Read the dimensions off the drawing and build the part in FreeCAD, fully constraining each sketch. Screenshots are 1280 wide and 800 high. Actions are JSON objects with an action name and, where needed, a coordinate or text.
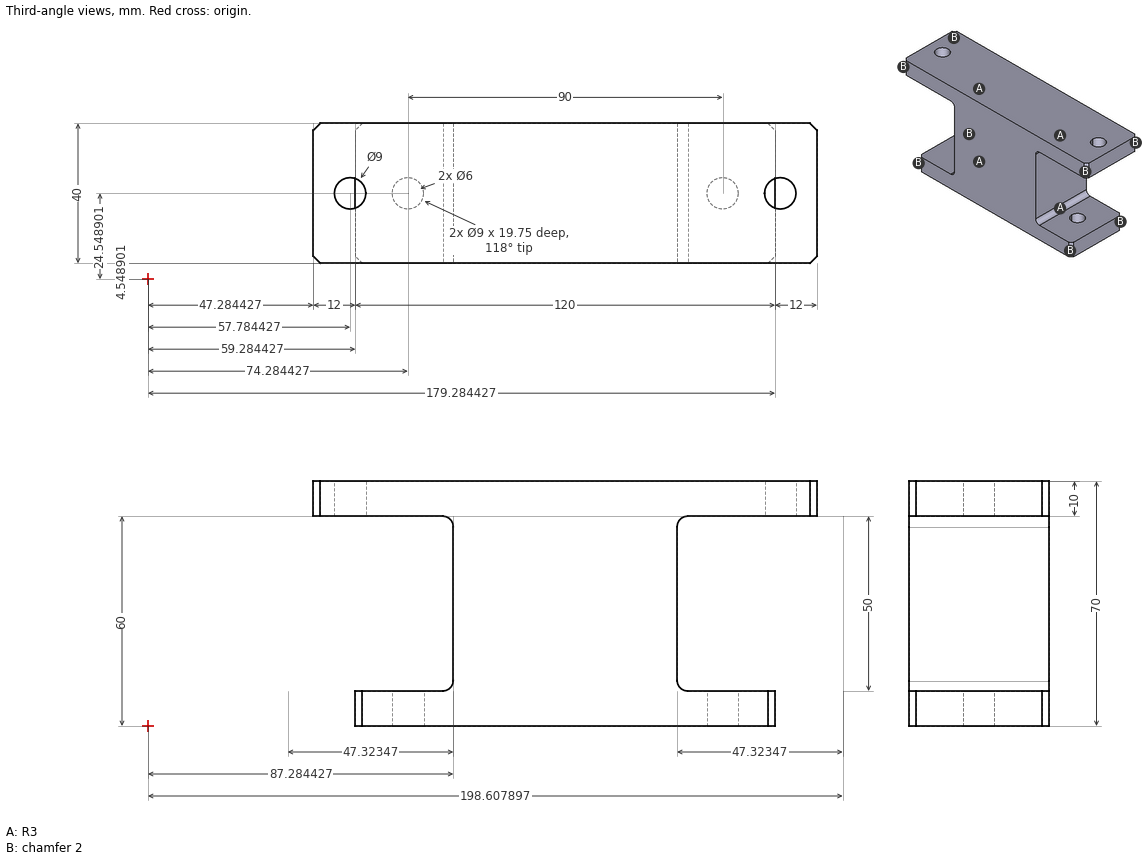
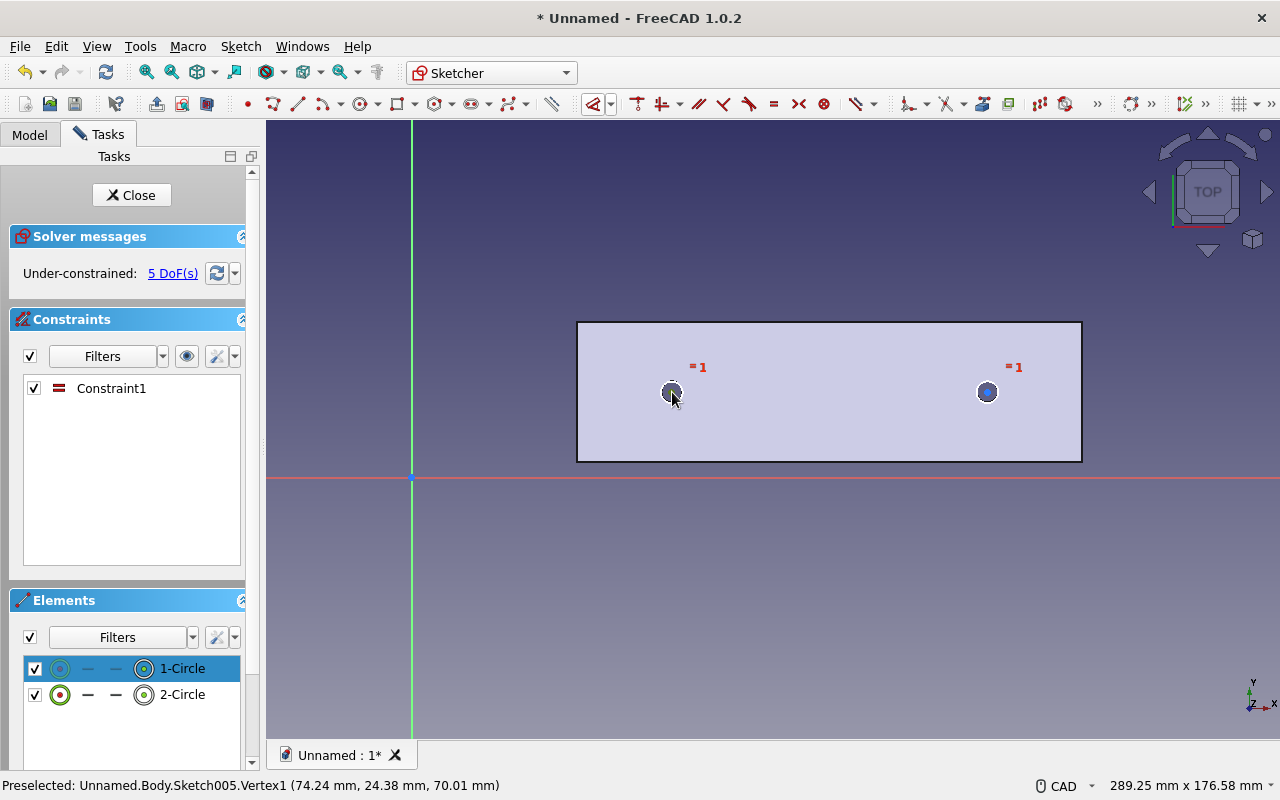
{"action": "left_click", "coordinate": [987, 392]}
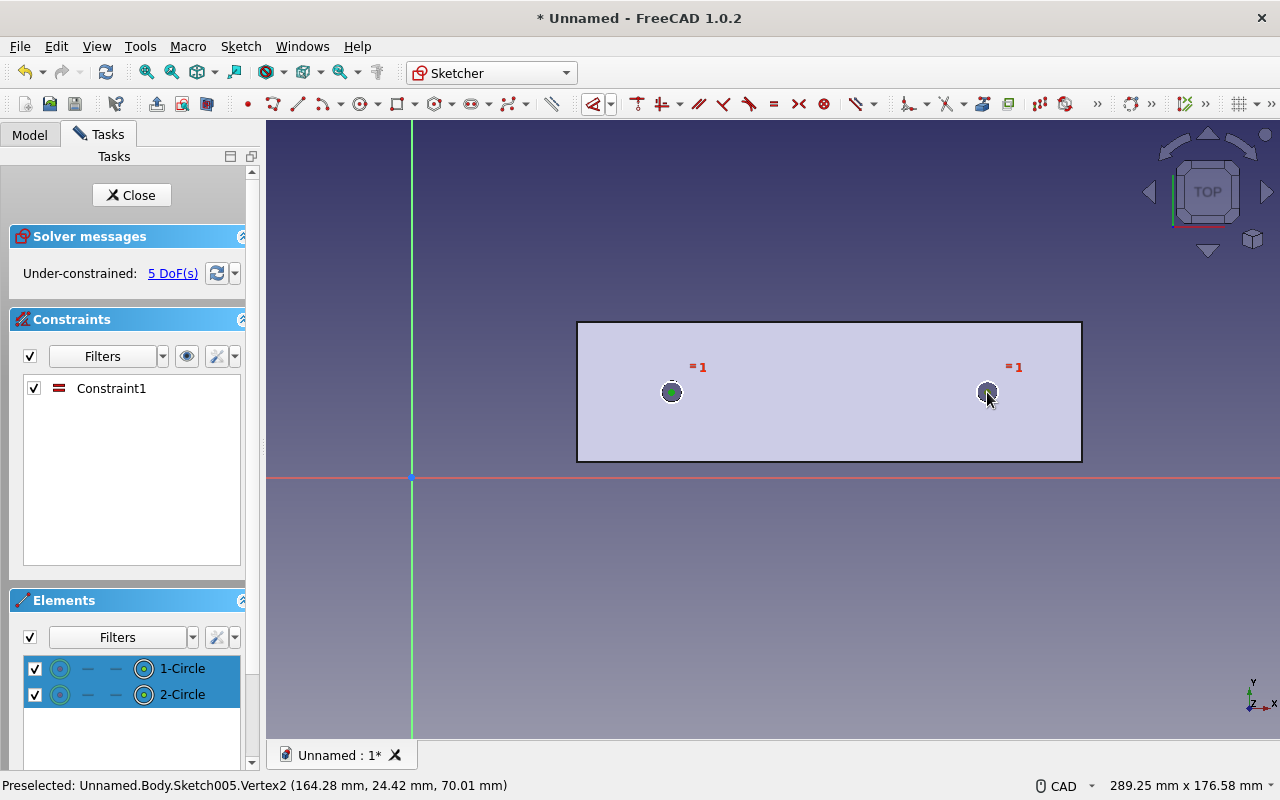
{"action": "key", "text": "h"}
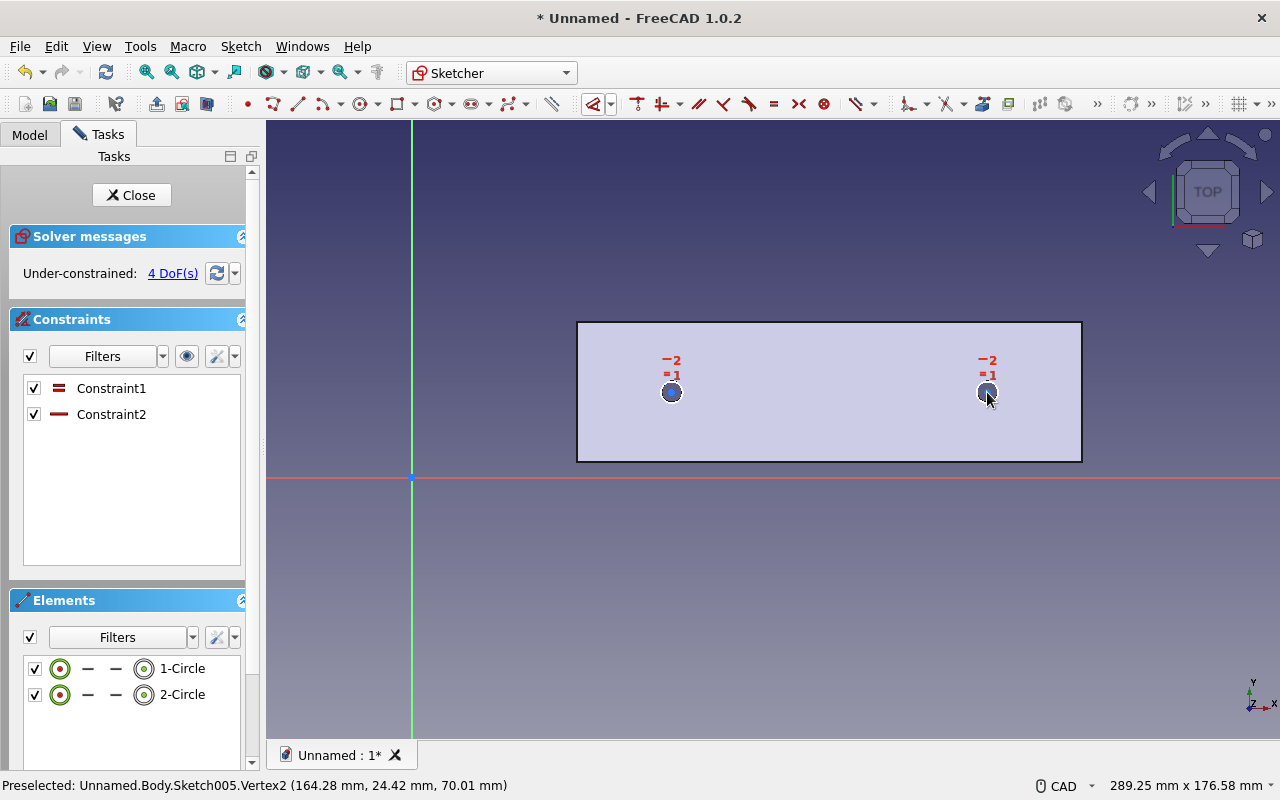
{"action": "scroll", "coordinate": [679, 385], "scroll_direction": "up", "scroll_amount": 4}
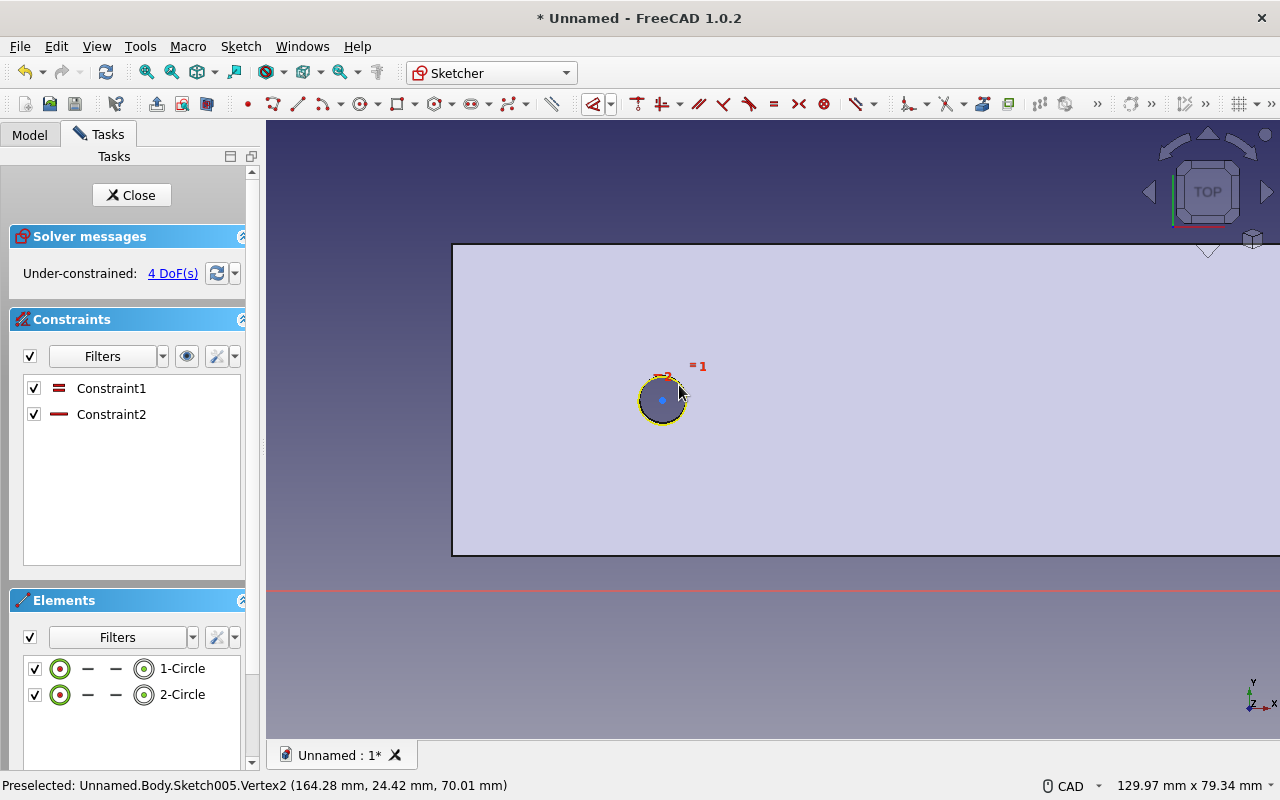
{"action": "left_click", "coordinate": [679, 384]}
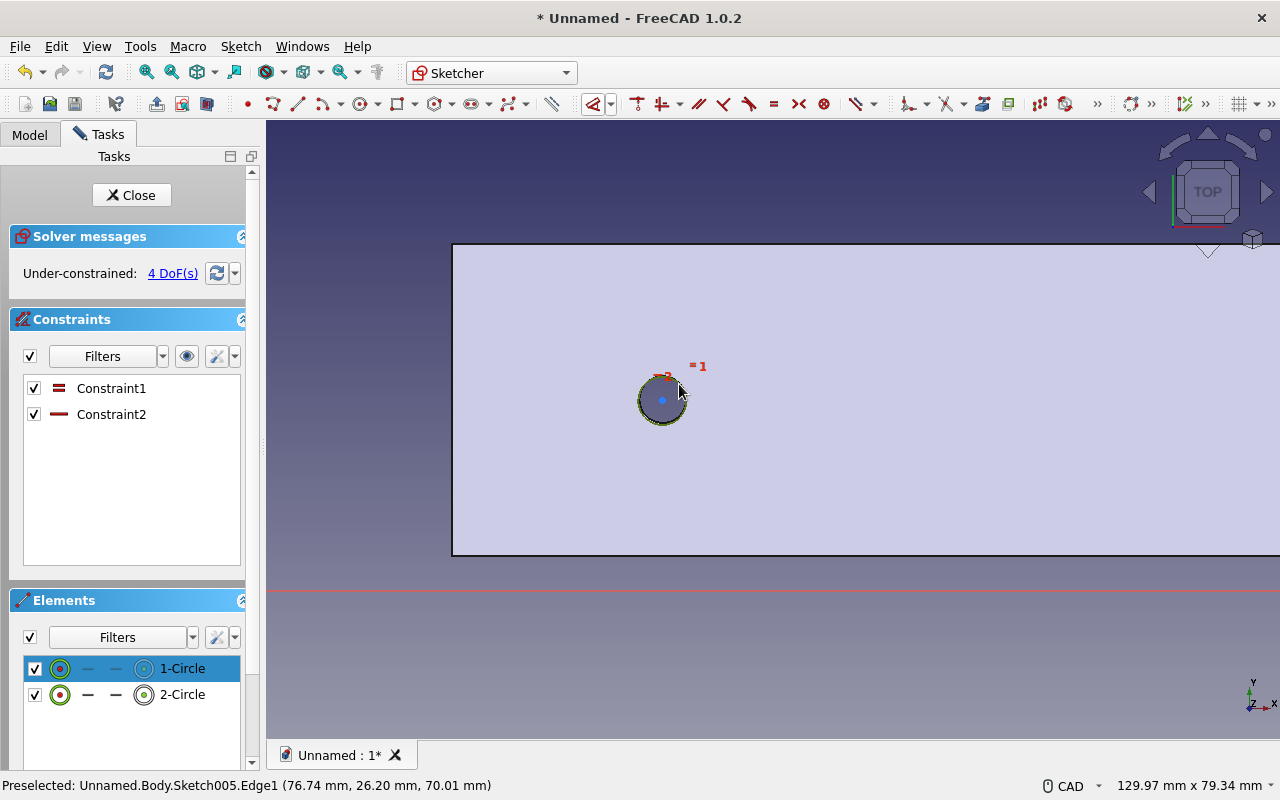
{"action": "key", "text": "k o"}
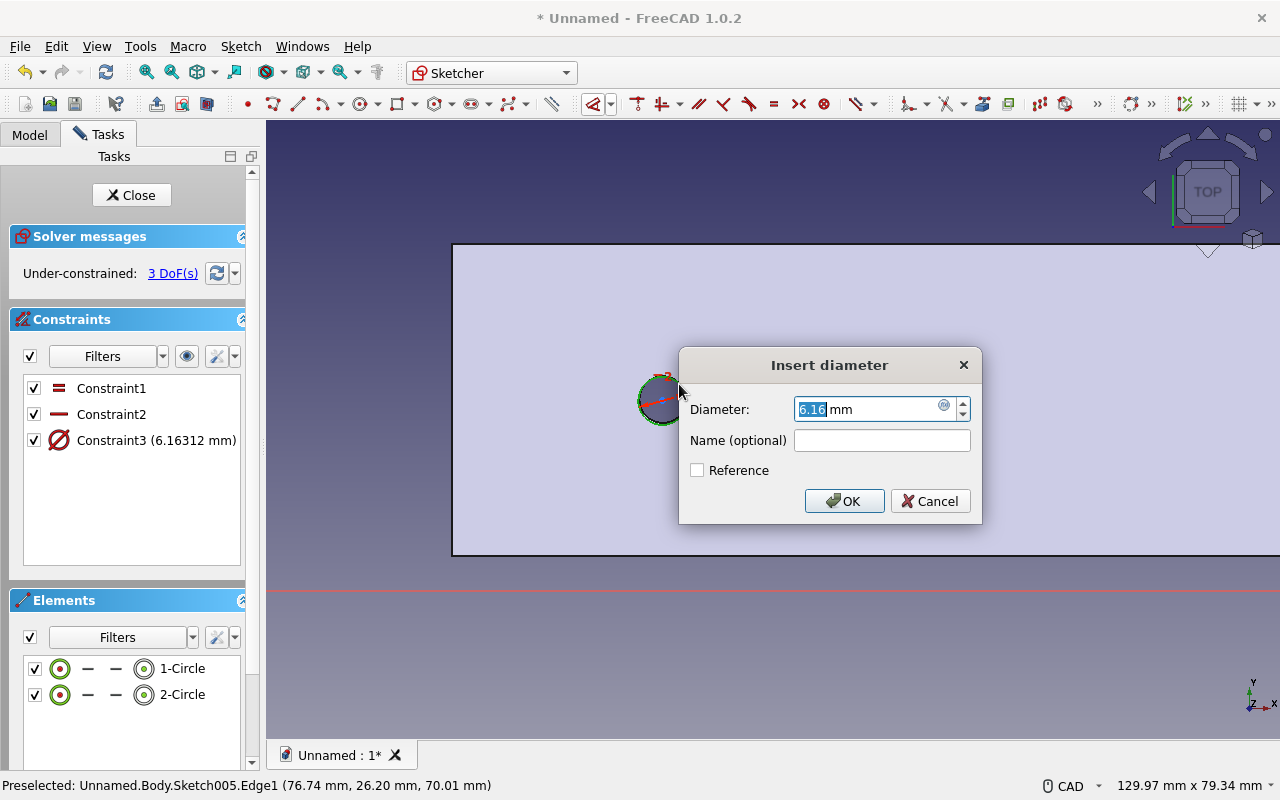
{"action": "type", "text": "6"}
{"action": "key", "text": "Return"}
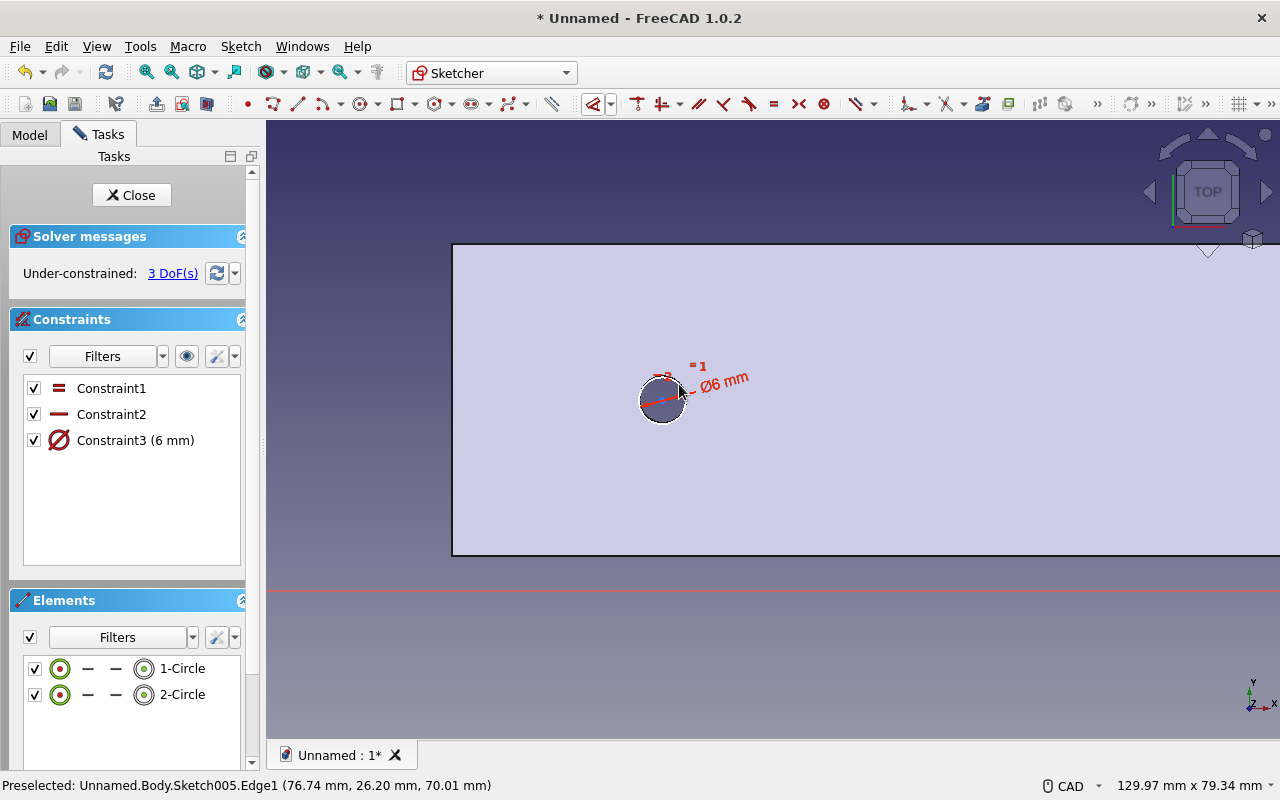
{"action": "left_click", "coordinate": [662, 401]}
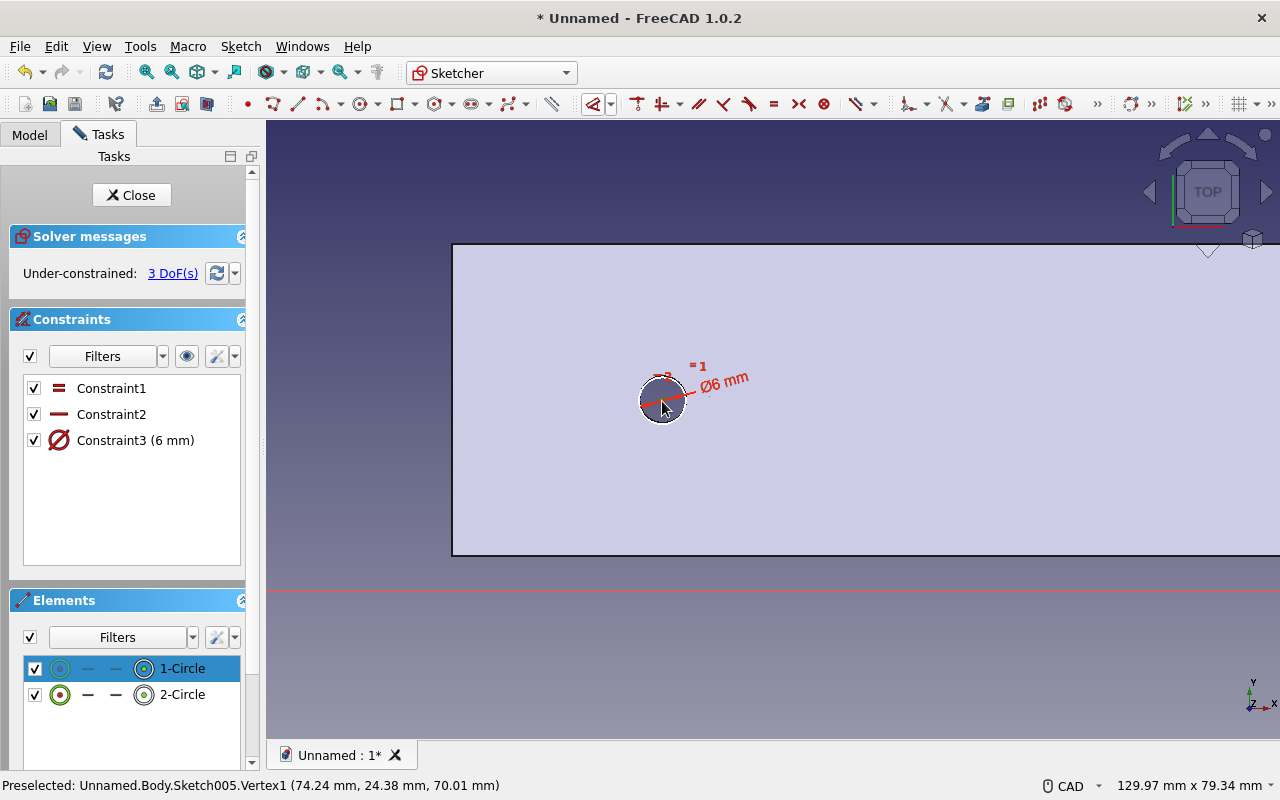
{"action": "scroll", "coordinate": [679, 385], "scroll_direction": "down", "scroll_amount": 4}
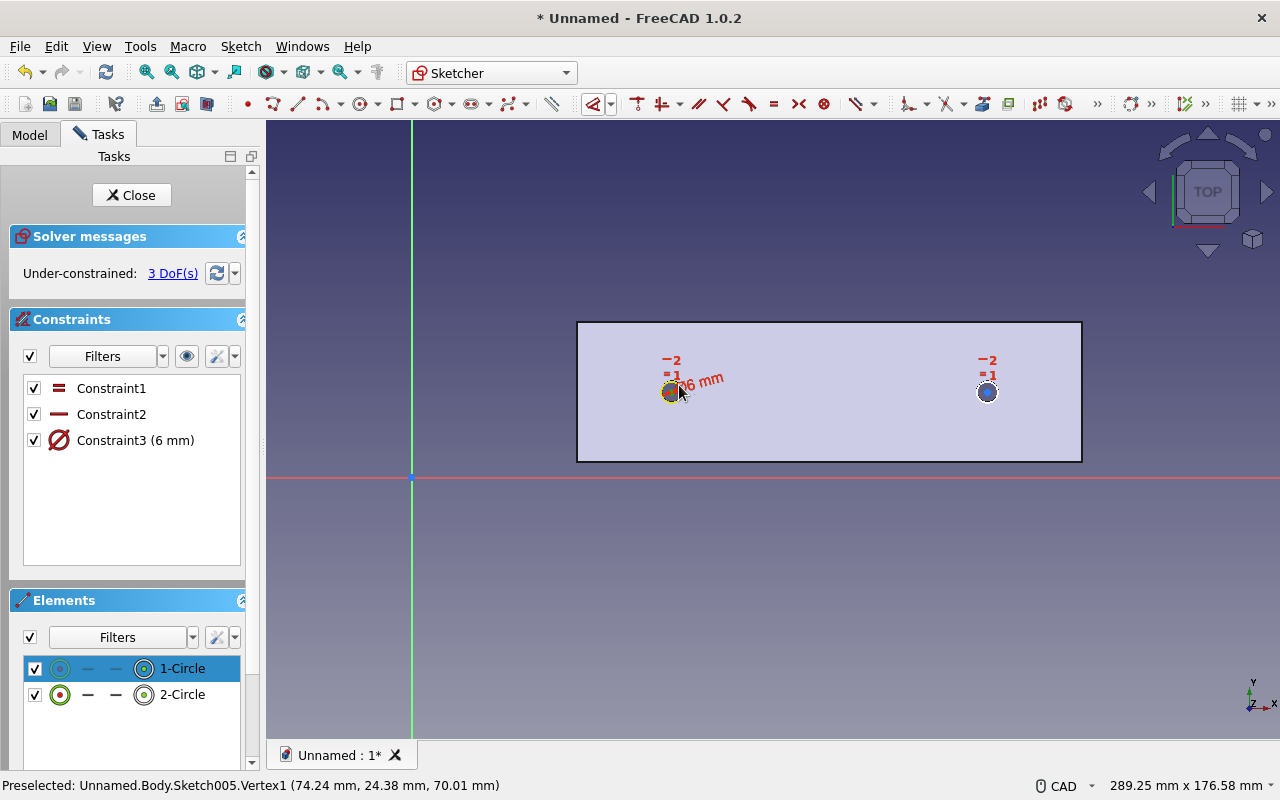
{"action": "left_click", "coordinate": [987, 392]}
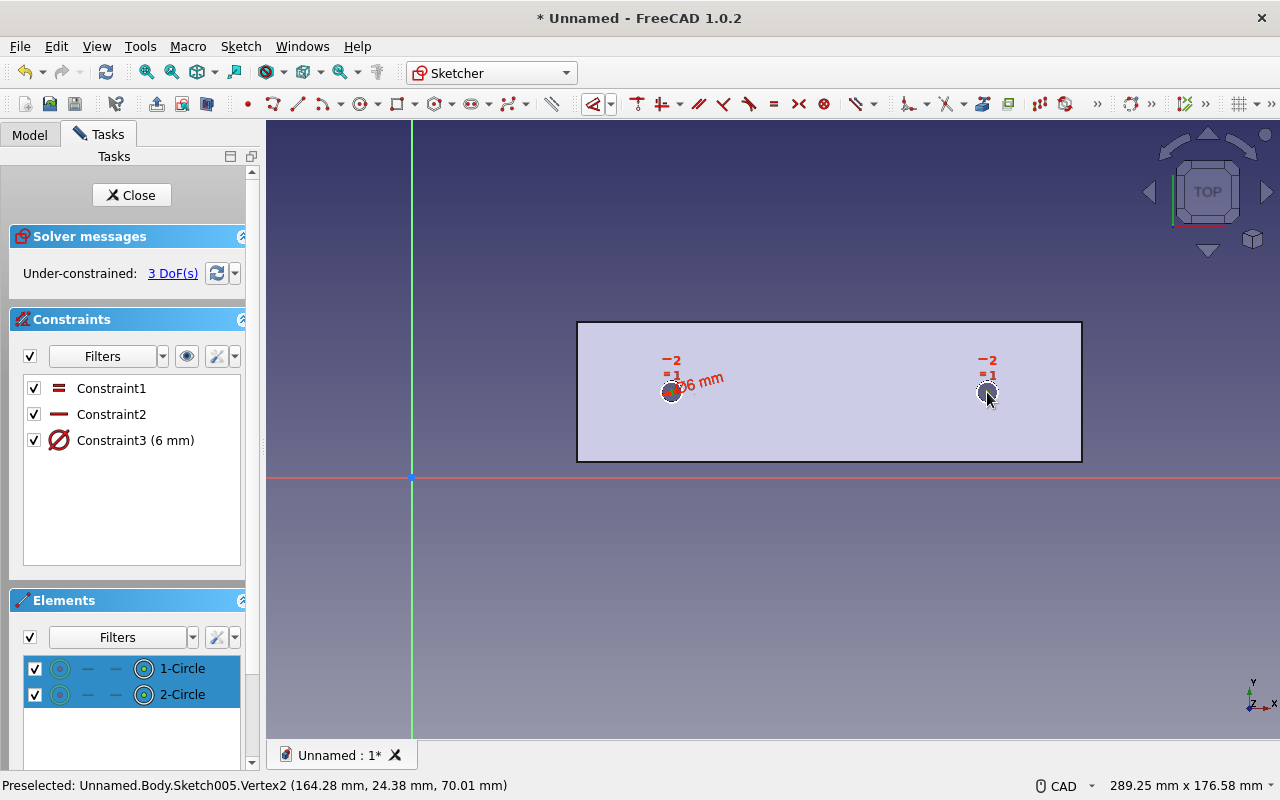
{"action": "key", "text": "l"}